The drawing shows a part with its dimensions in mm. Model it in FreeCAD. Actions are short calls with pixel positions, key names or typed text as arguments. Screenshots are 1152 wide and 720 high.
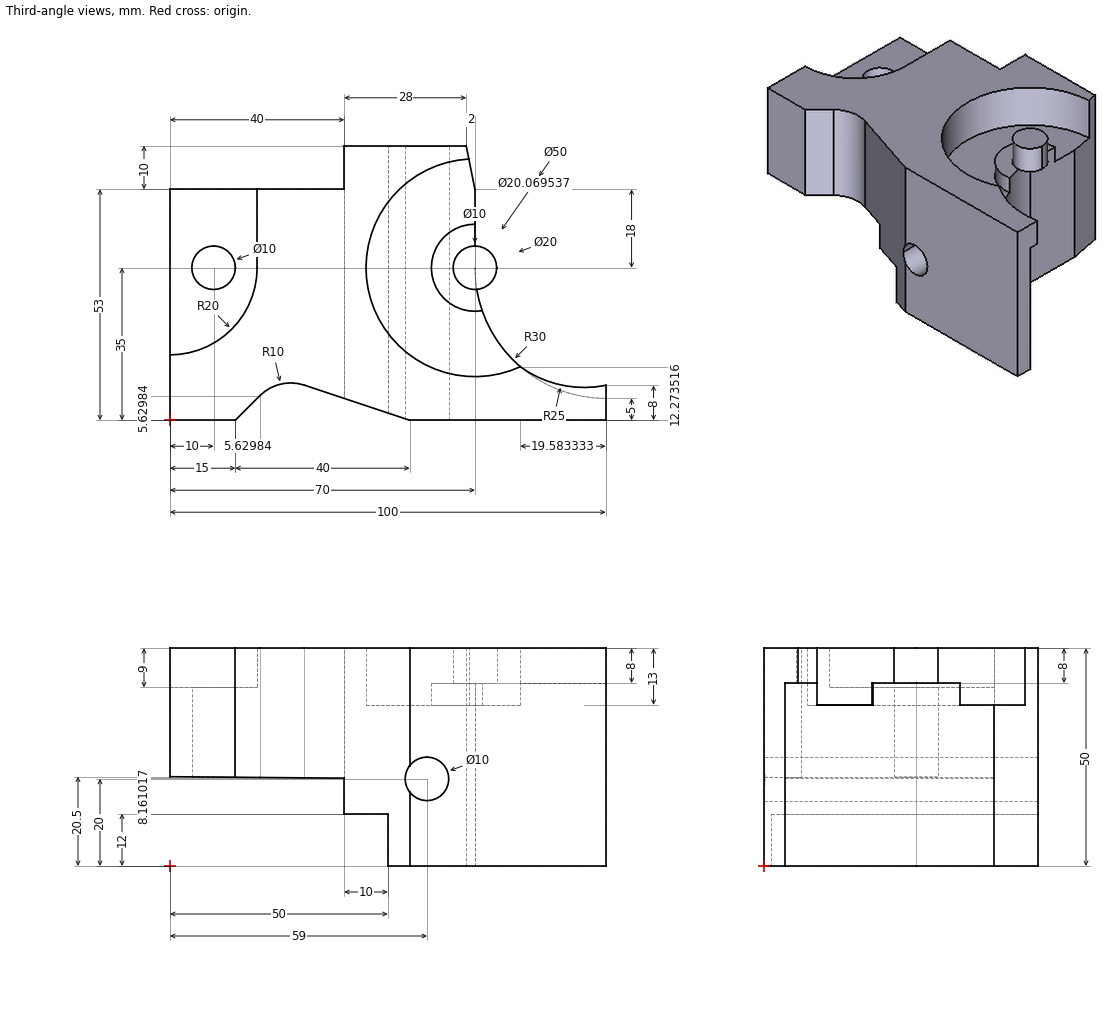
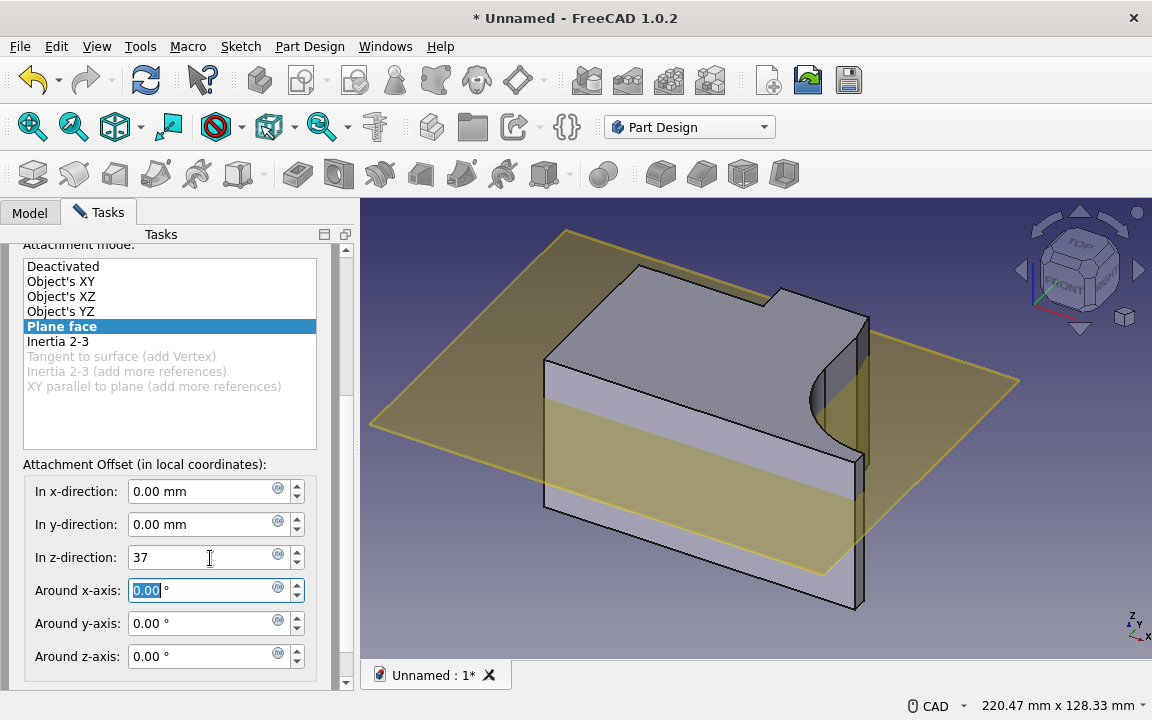
scroll(346, 467, up, 5)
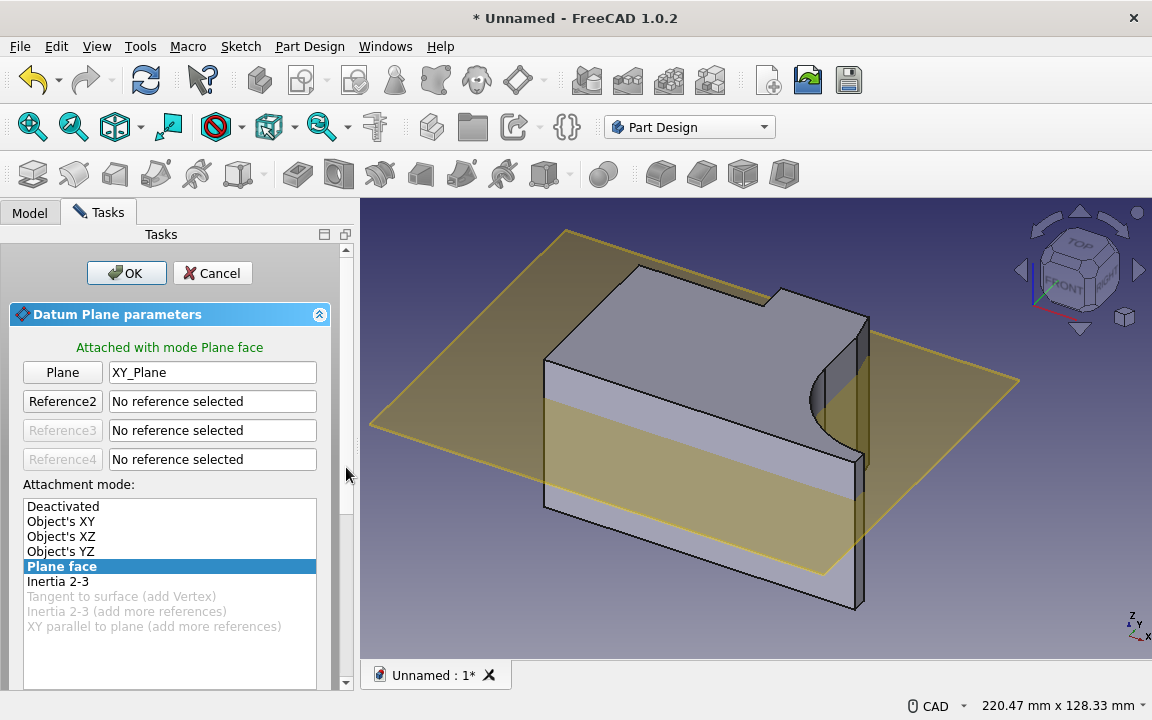
click(127, 273)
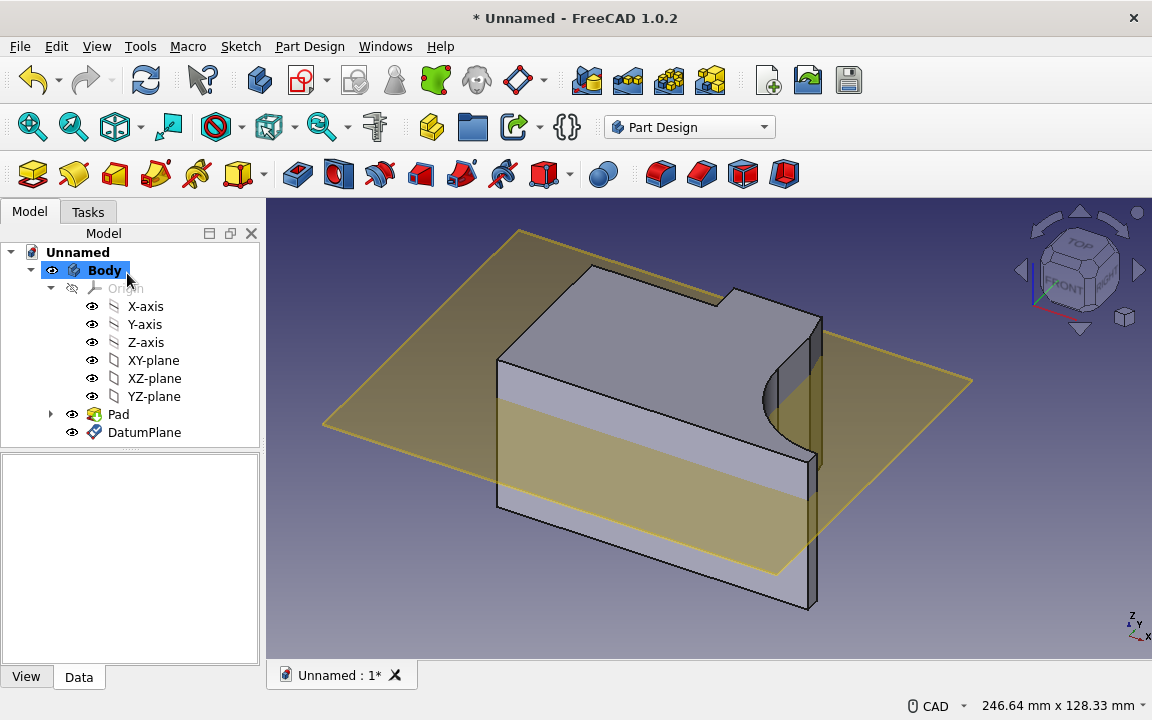
click(117, 432)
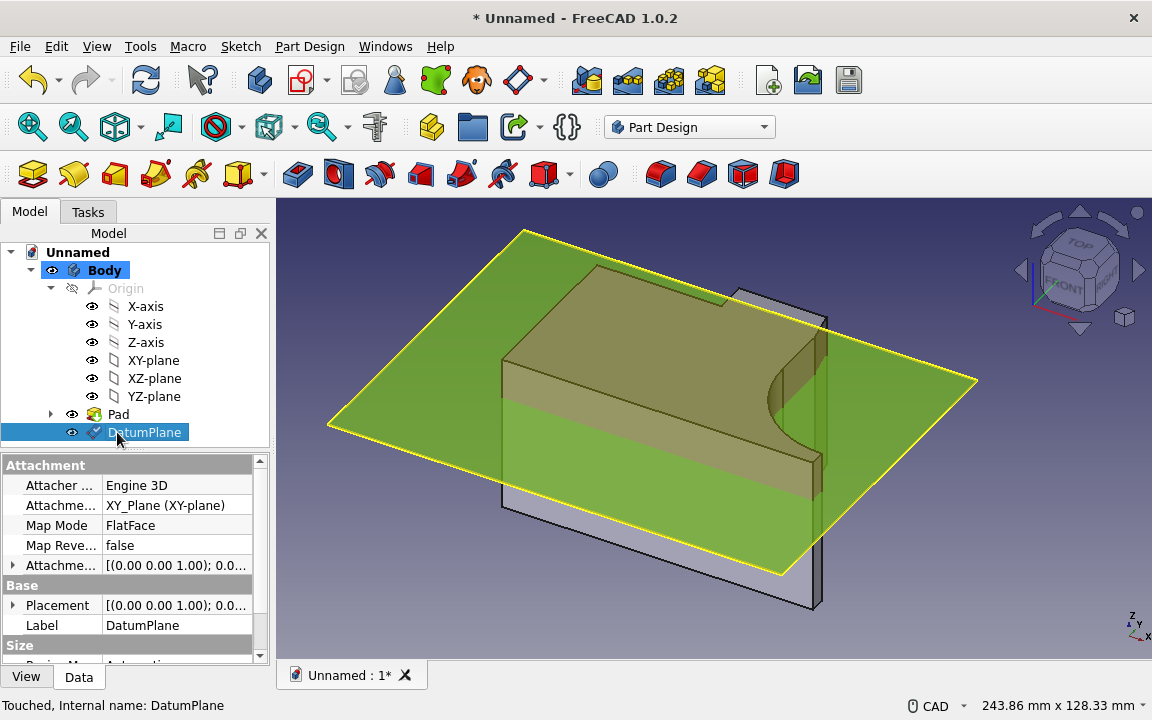
click(300, 80)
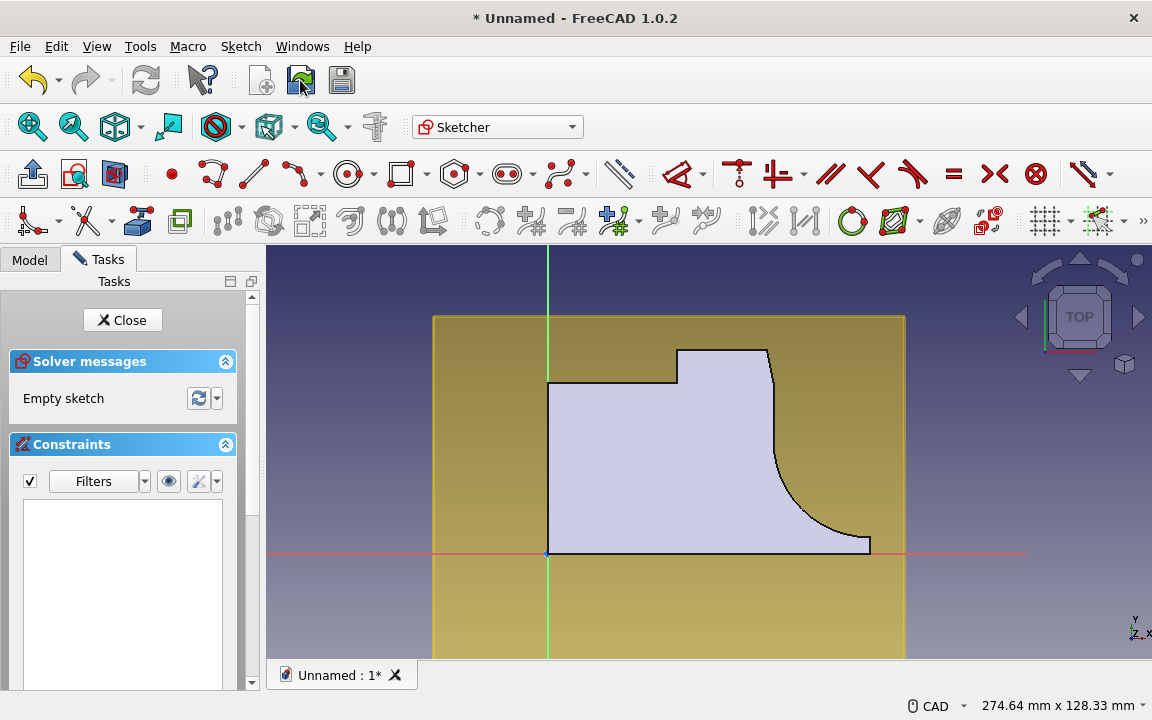
key(q)
key(s)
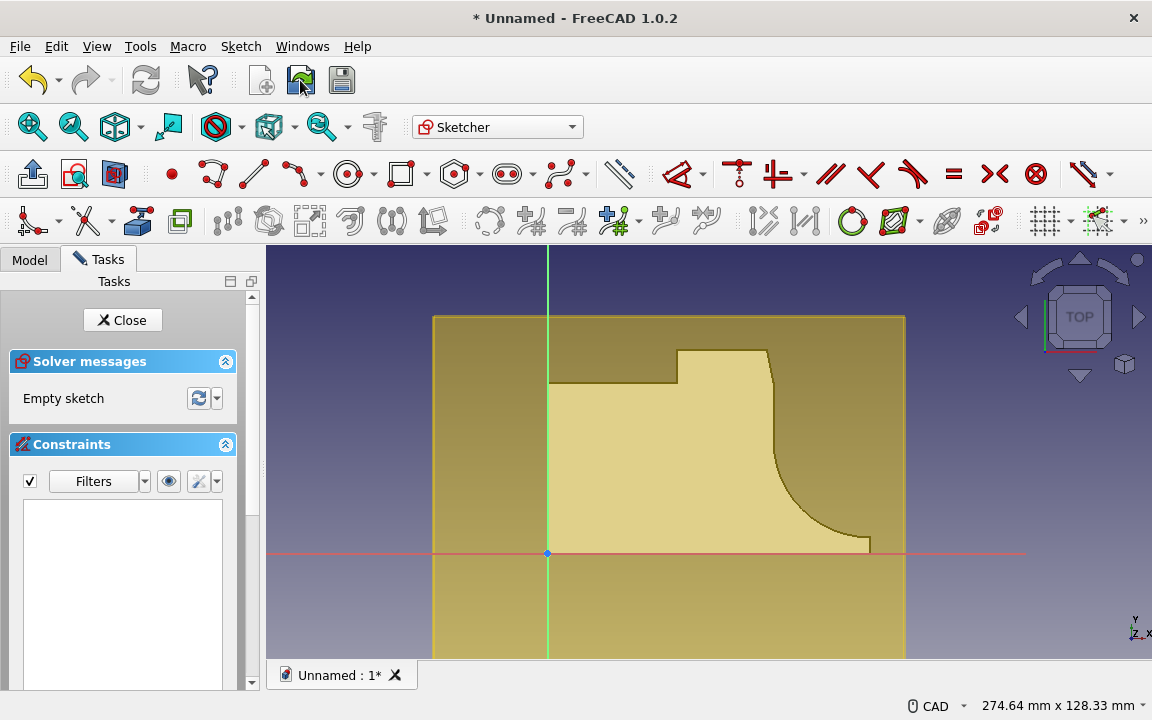
key(g)
key(c)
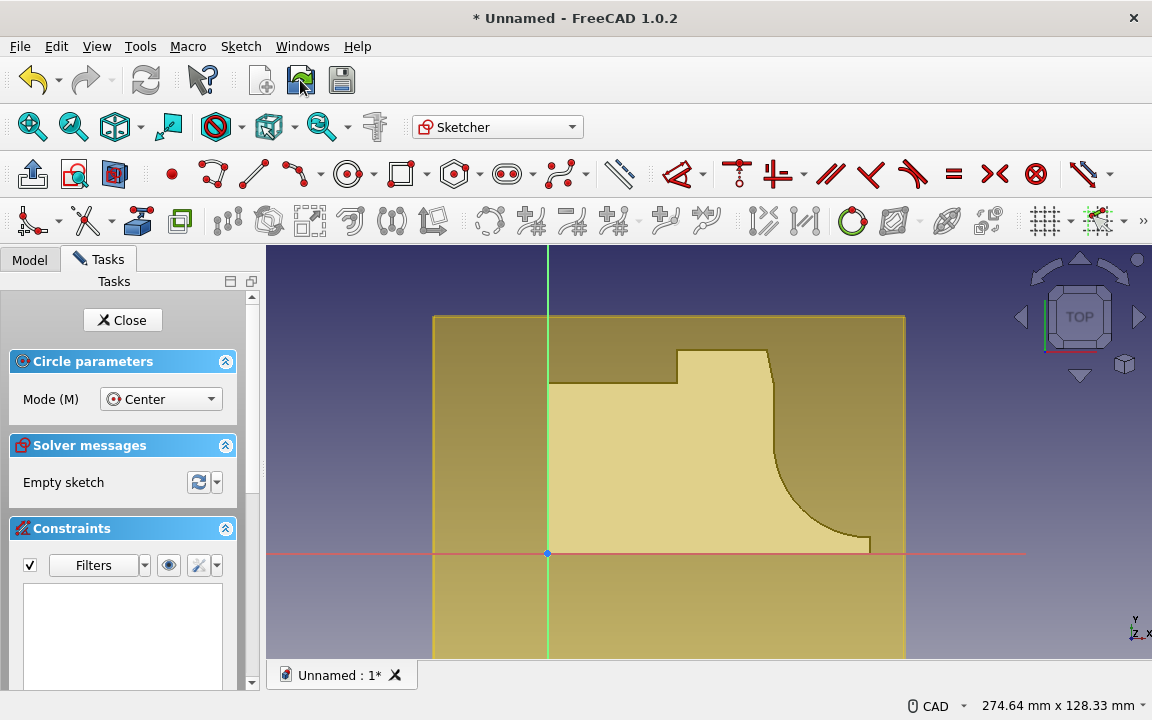
click(774, 441)
click(831, 384)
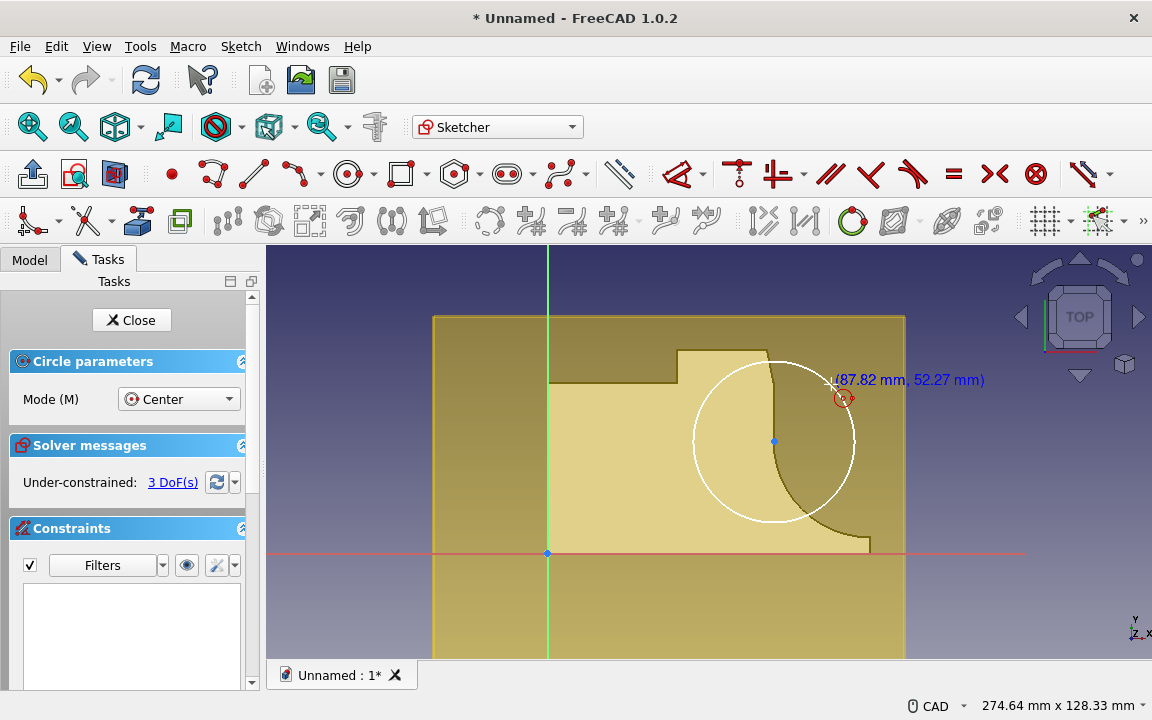
click(774, 442)
click(796, 418)
key(Escape)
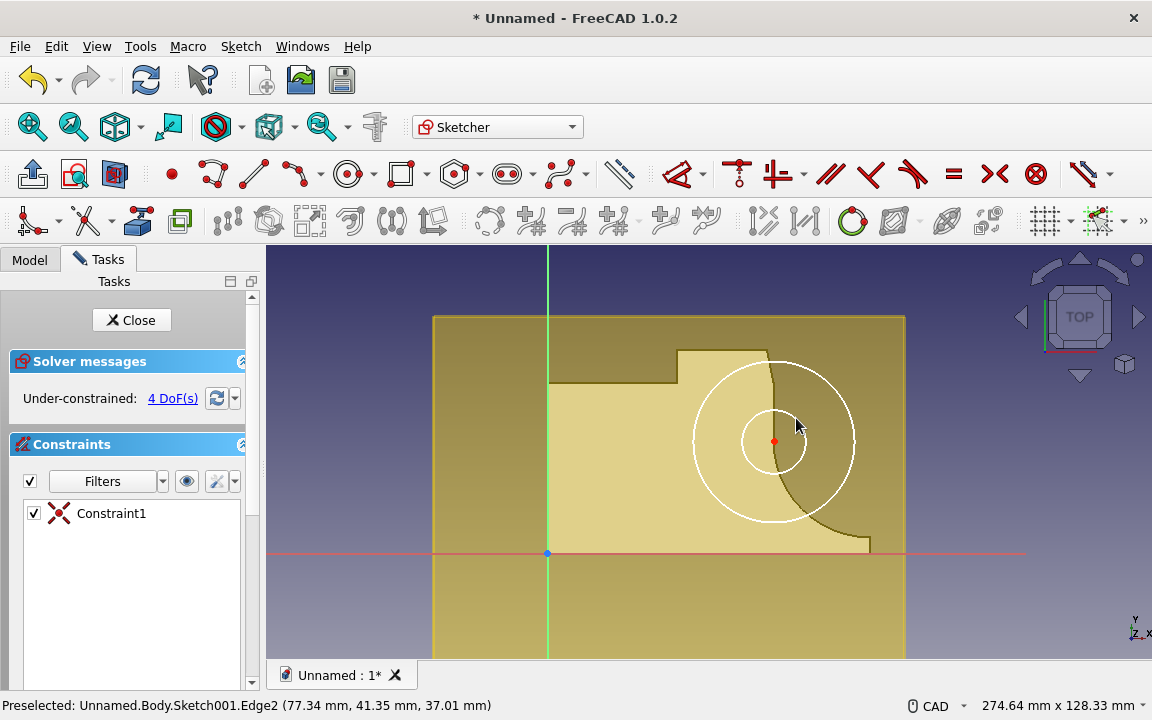
key(d)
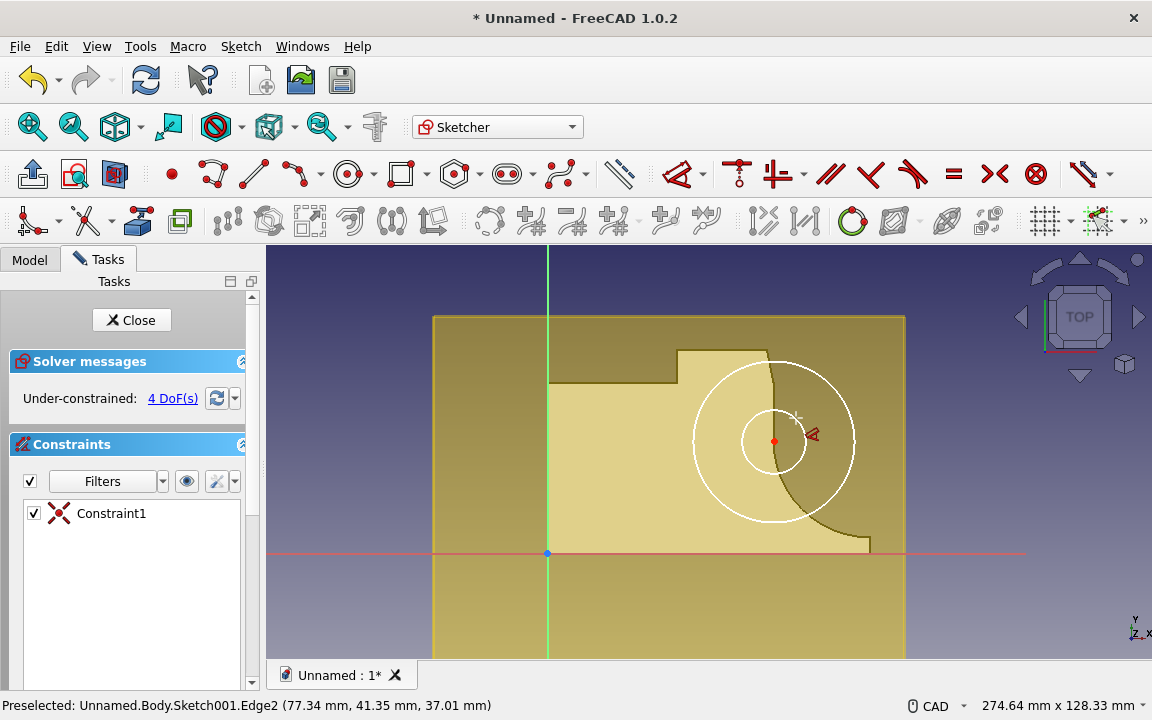
click(831, 385)
click(854, 362)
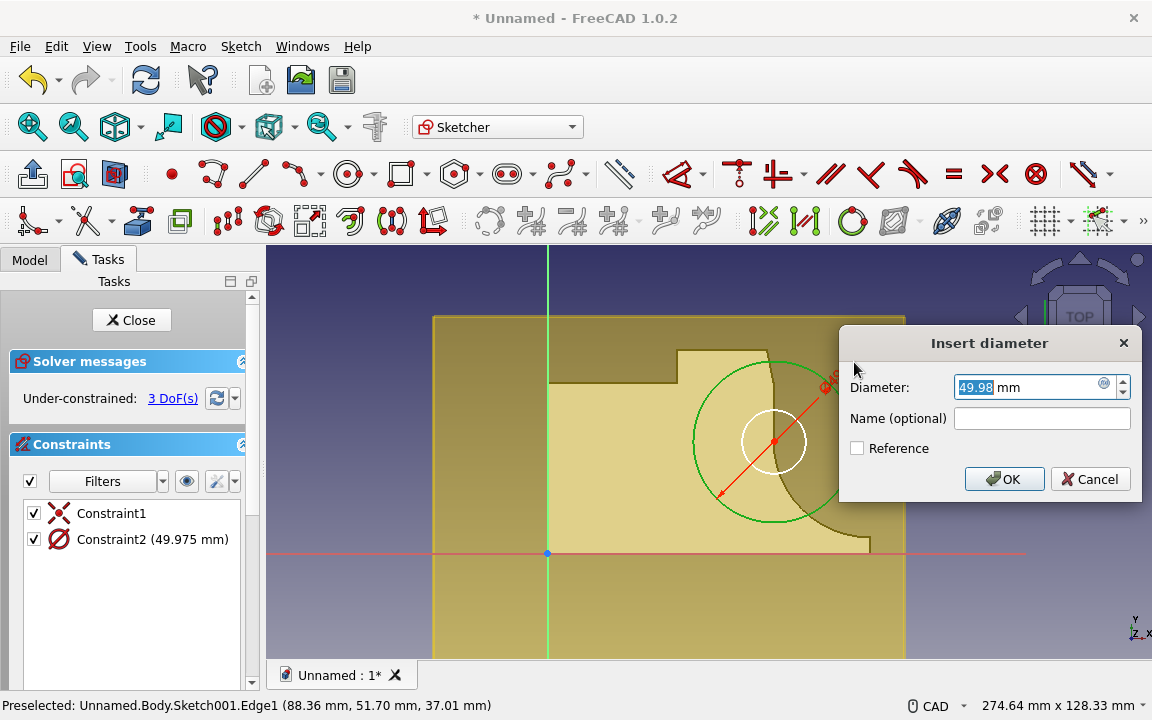
text(50)
key(Return)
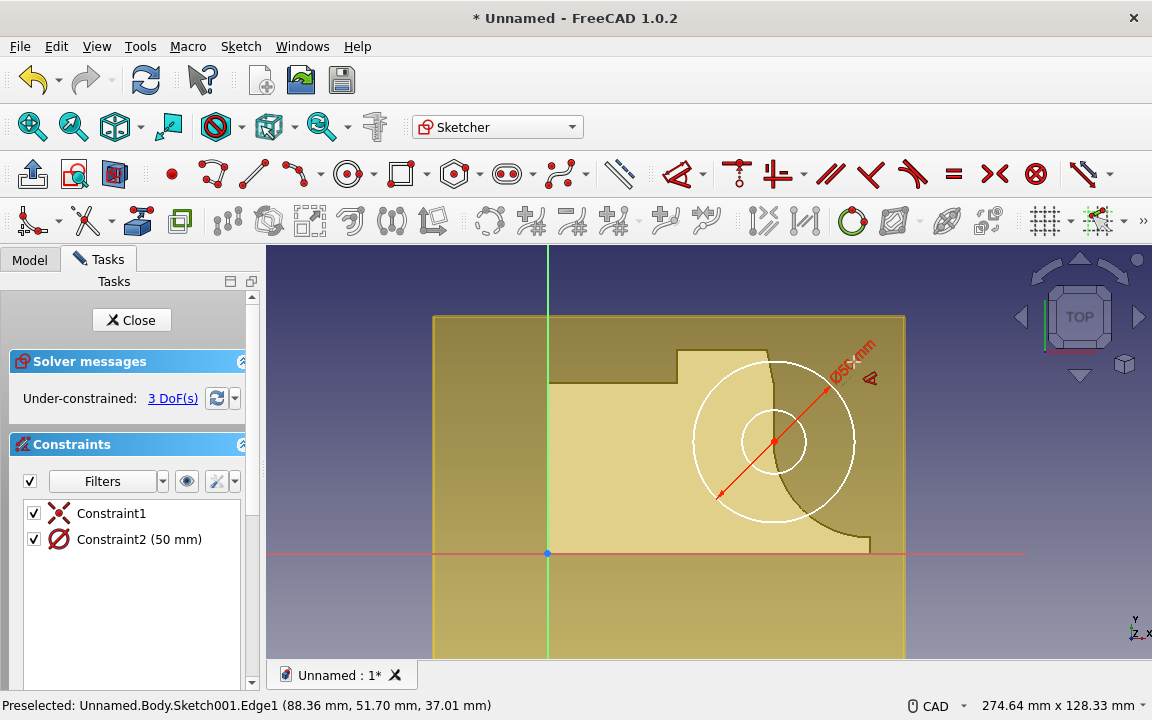
click(796, 419)
click(818, 396)